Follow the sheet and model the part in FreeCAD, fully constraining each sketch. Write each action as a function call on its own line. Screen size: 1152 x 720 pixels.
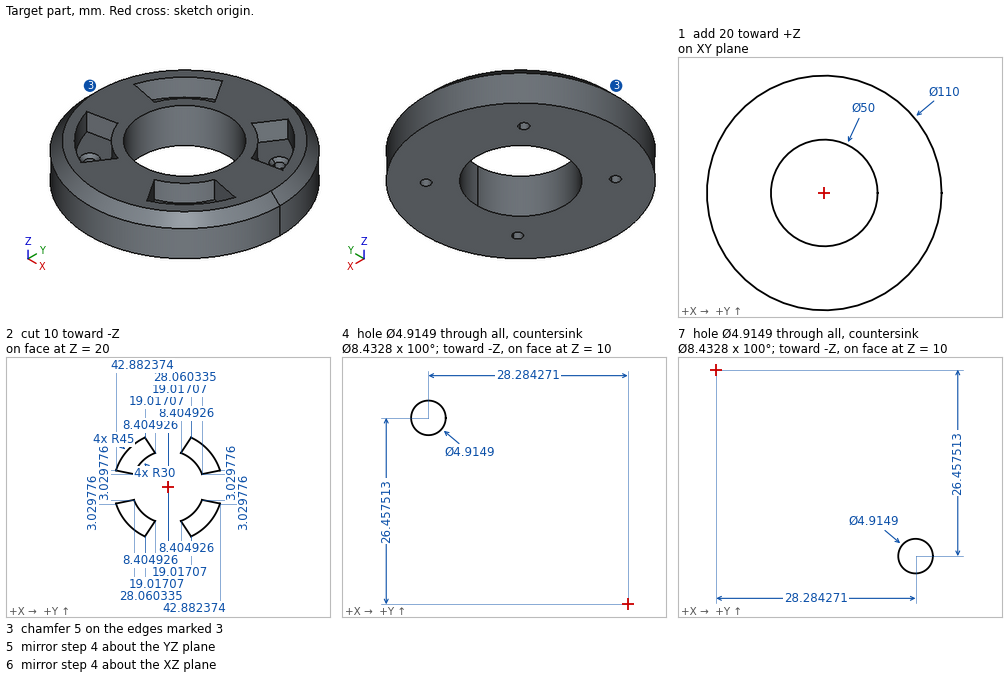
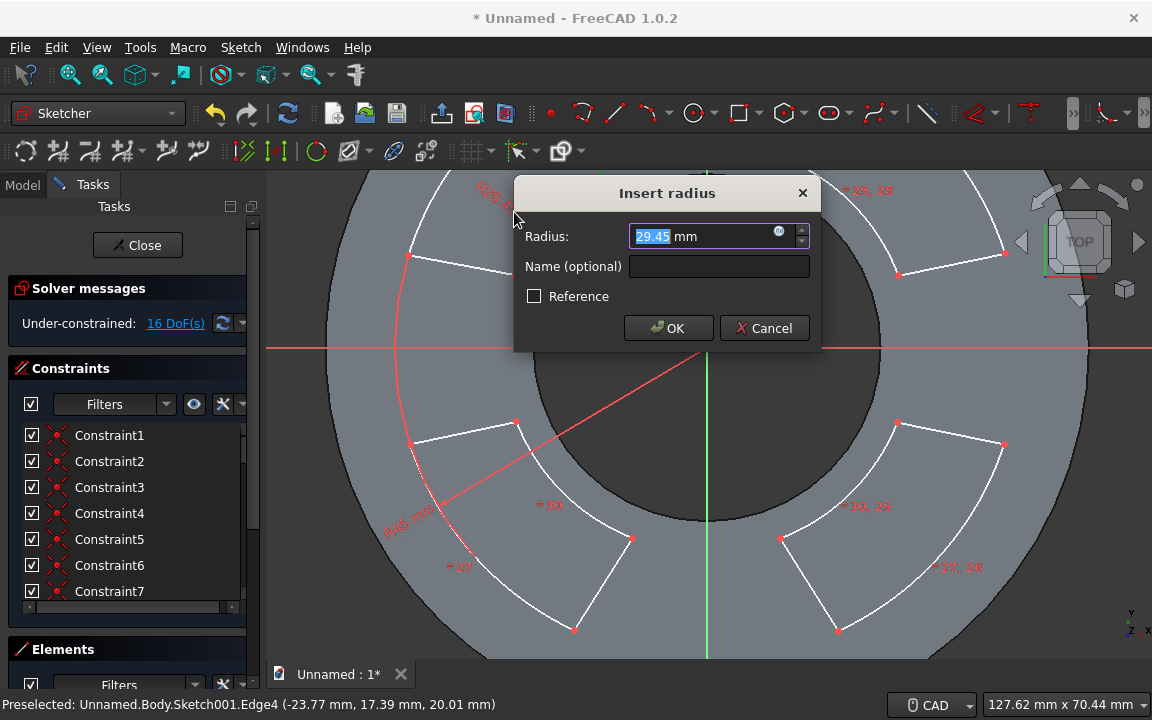
text(30)
key(Return)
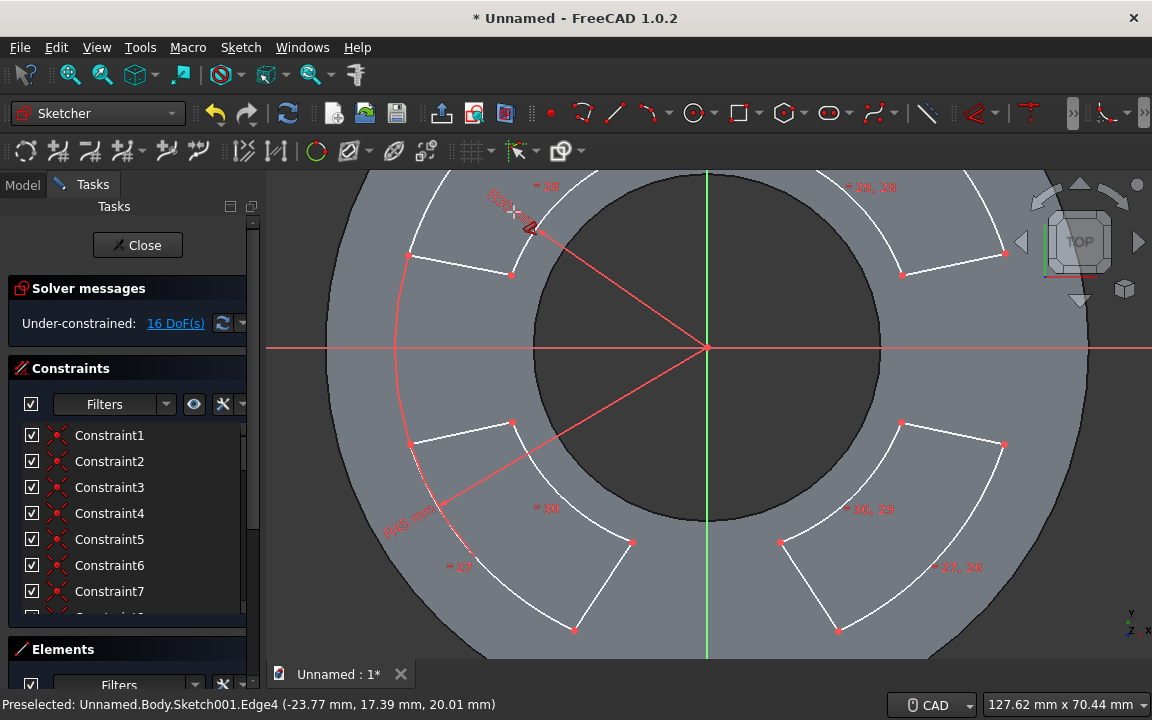
scroll(560, 496, down, 3)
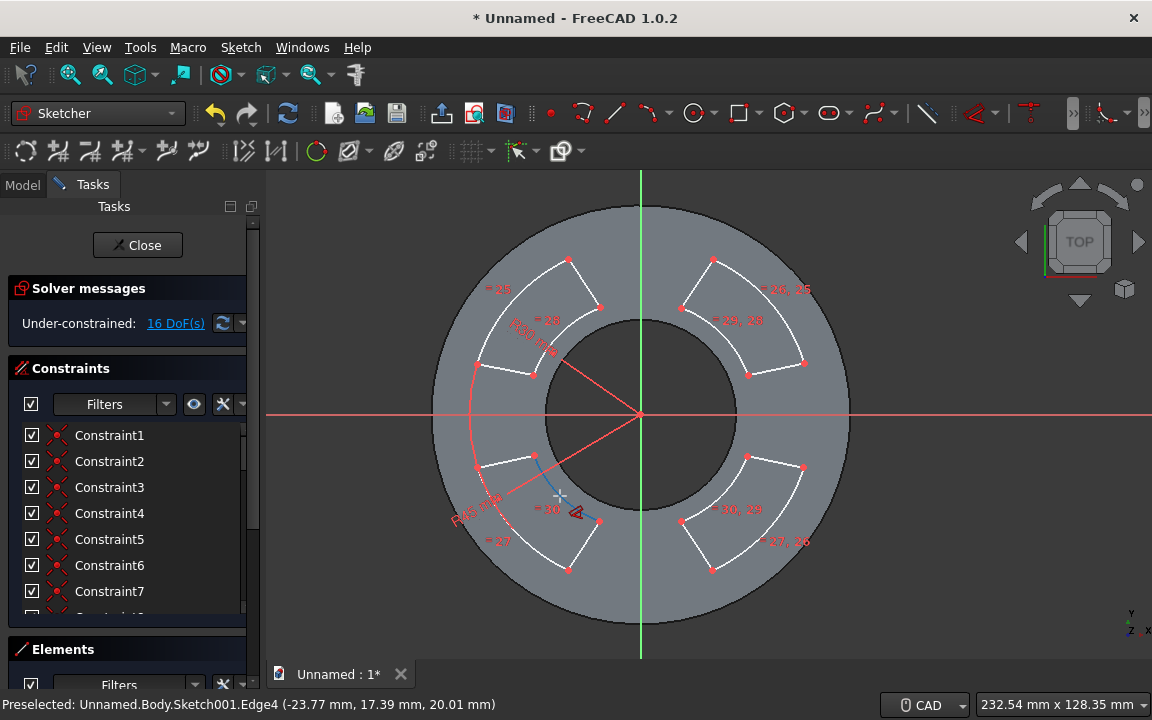
click(569, 259)
click(605, 225)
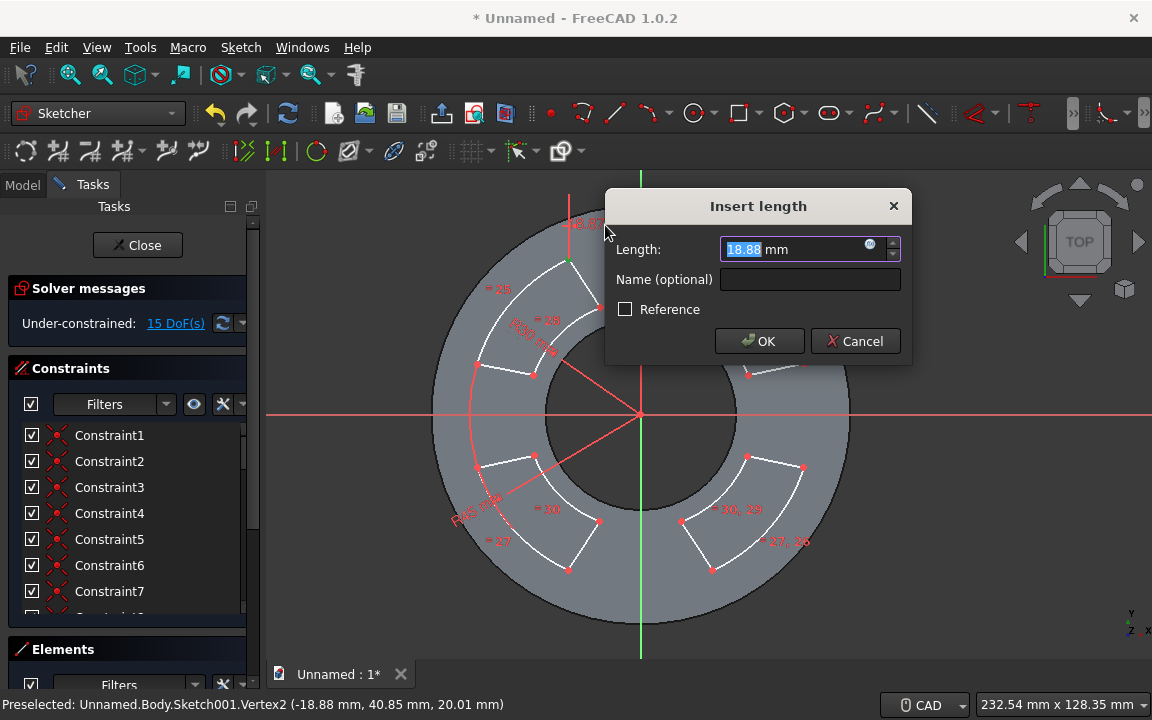
text(19.01707)
key(Return)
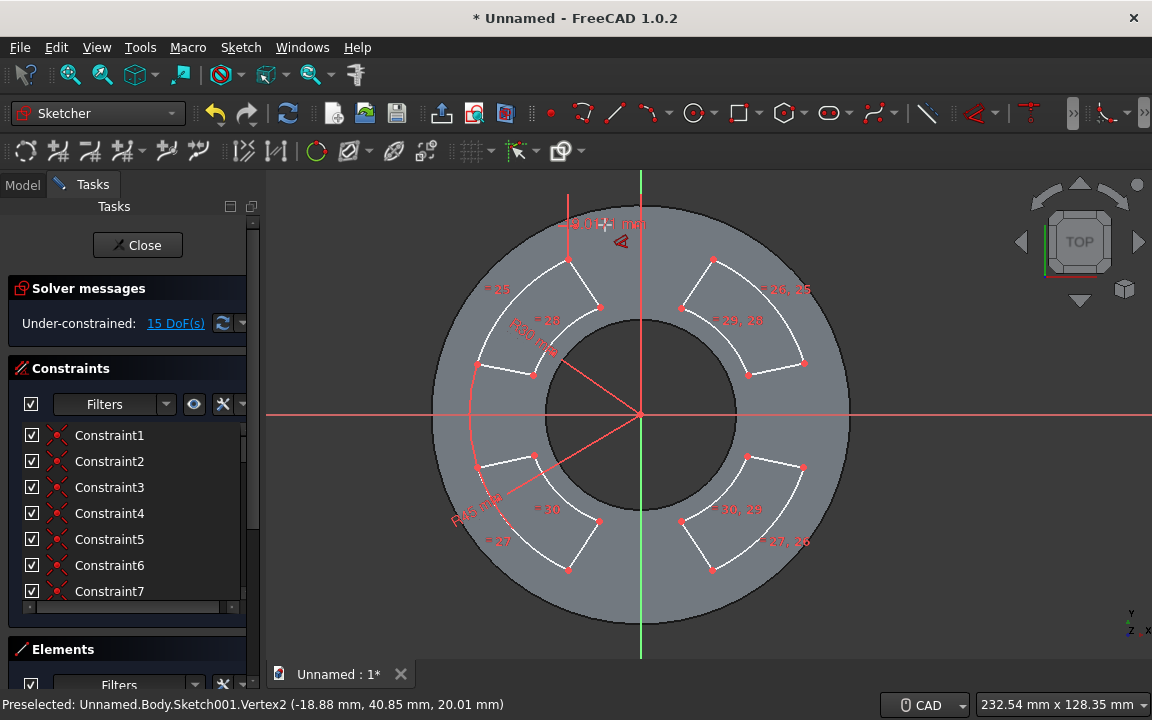
click(713, 260)
click(677, 226)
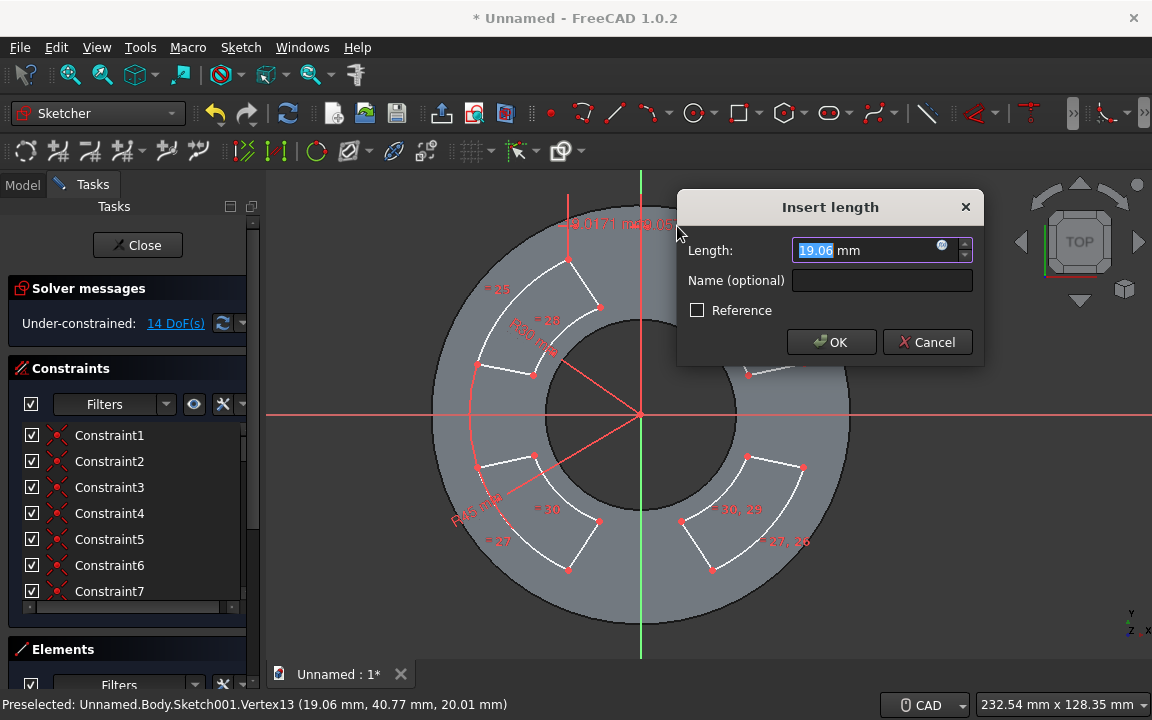
text(19.01707)
key(Return)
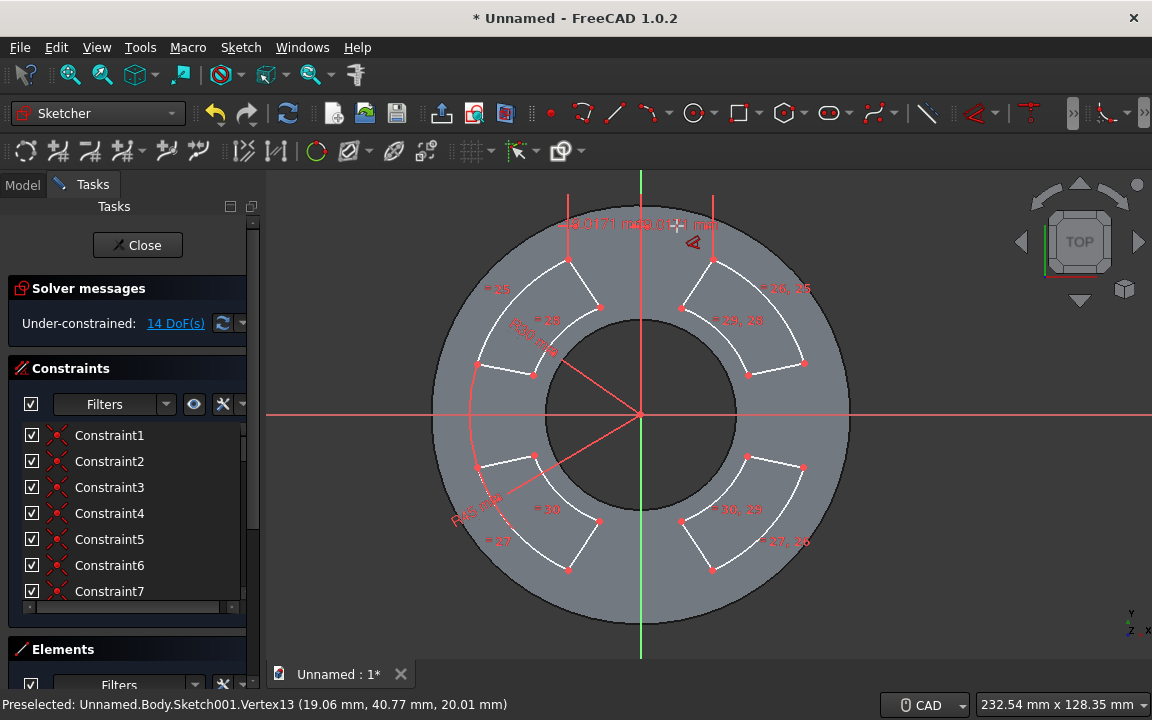
click(713, 570)
click(677, 604)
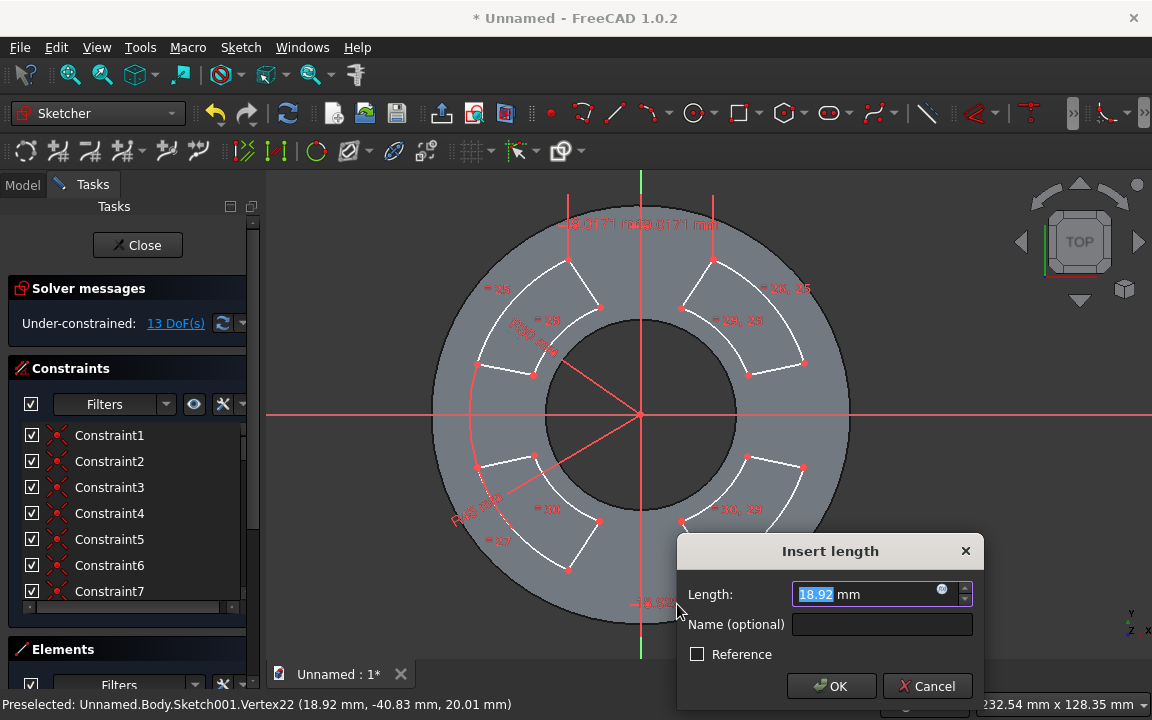
text(19.01707)
key(Return)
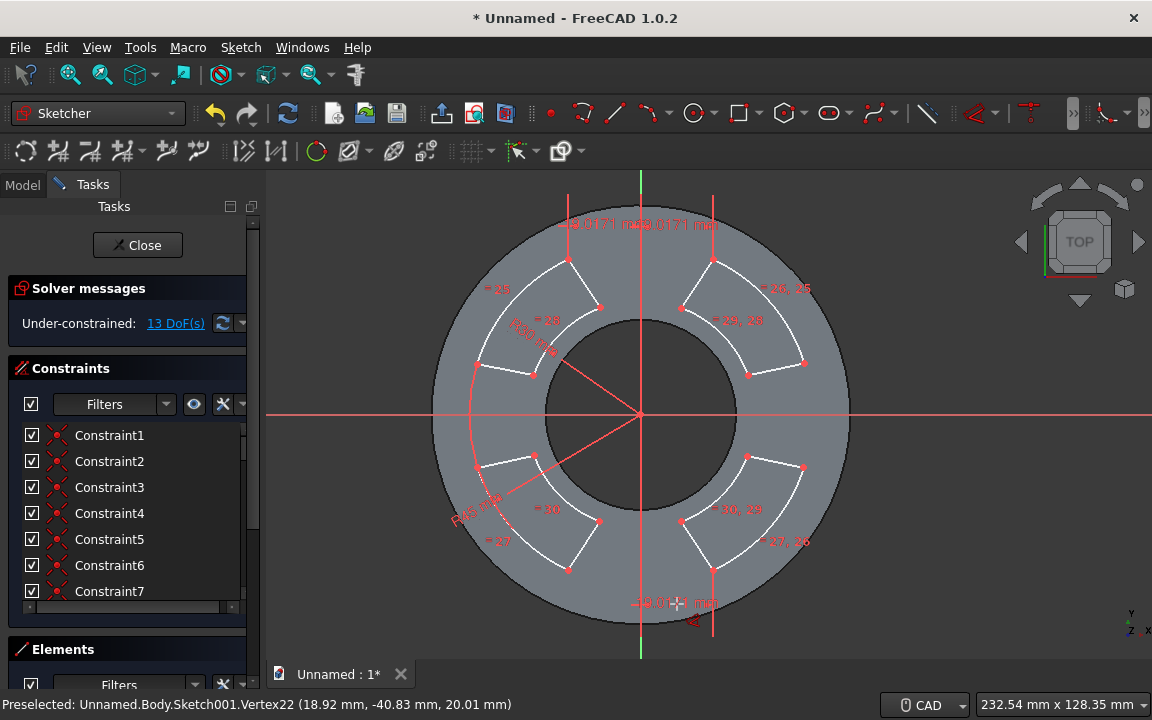
click(568, 570)
click(604, 604)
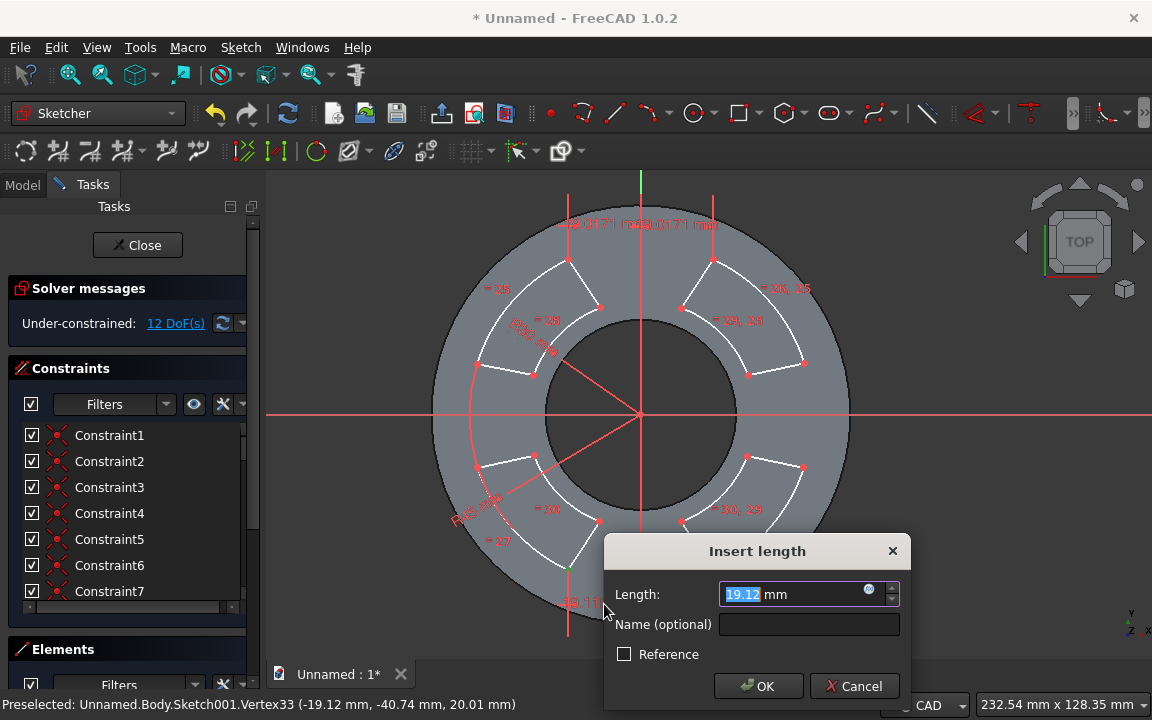
text(19.01707)
key(Return)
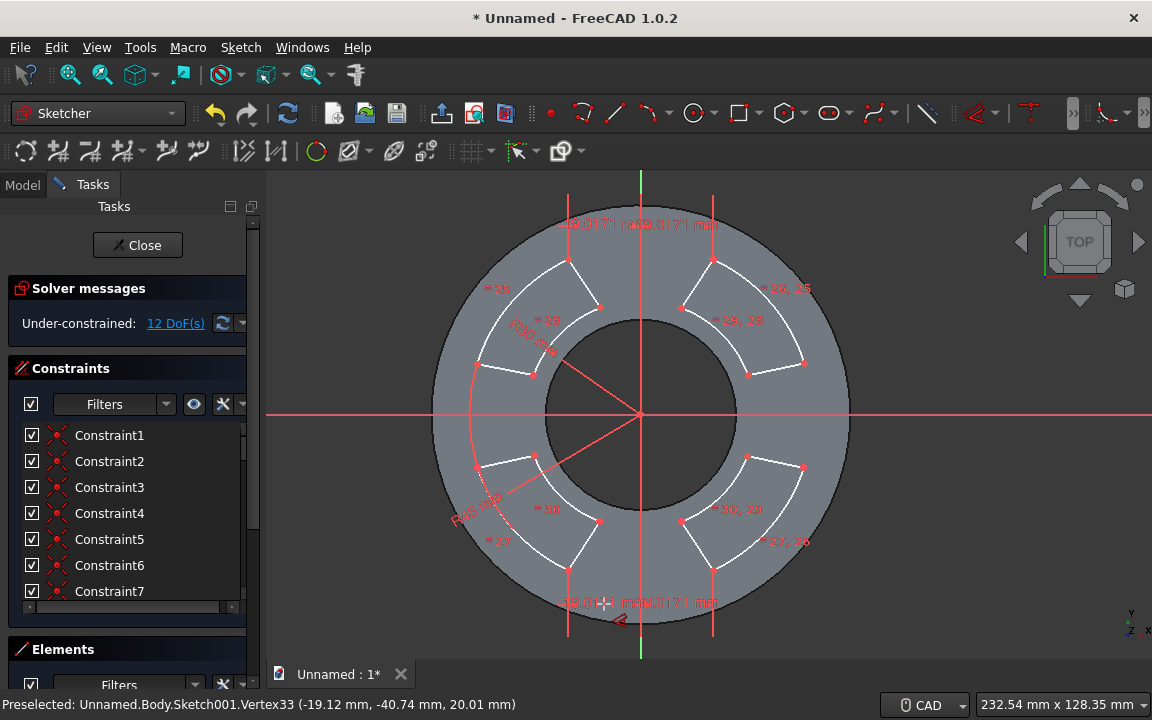
scroll(591, 293, up, 2)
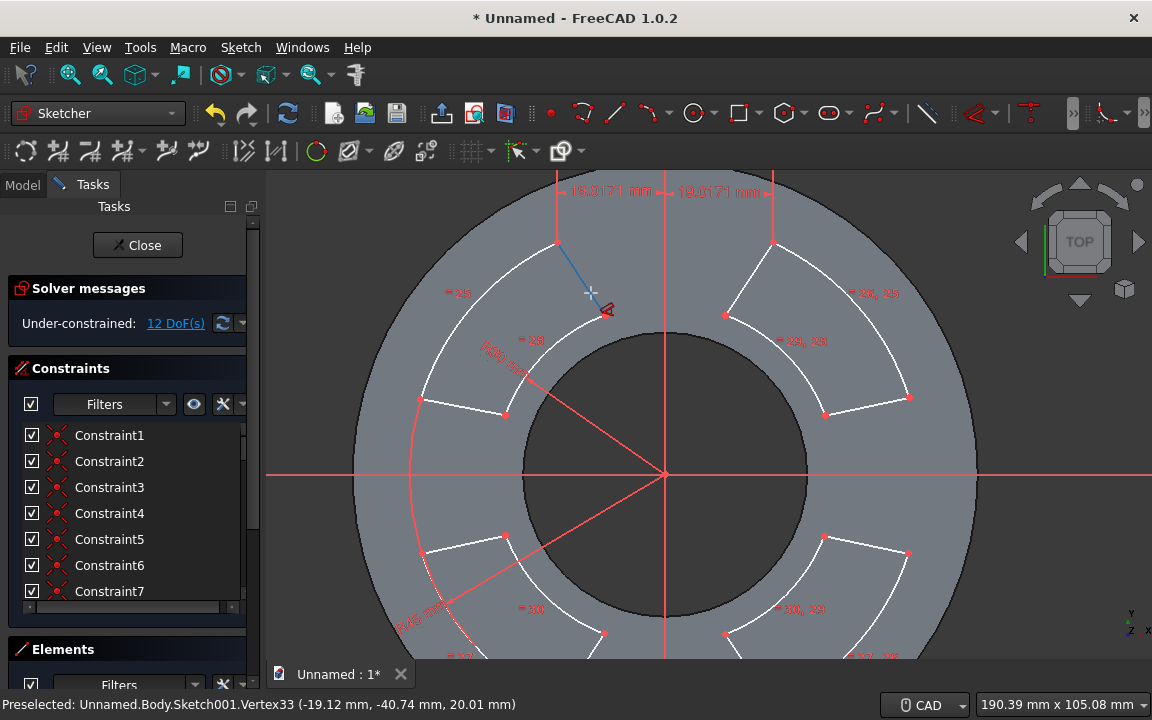
click(591, 293)
click(581, 349)